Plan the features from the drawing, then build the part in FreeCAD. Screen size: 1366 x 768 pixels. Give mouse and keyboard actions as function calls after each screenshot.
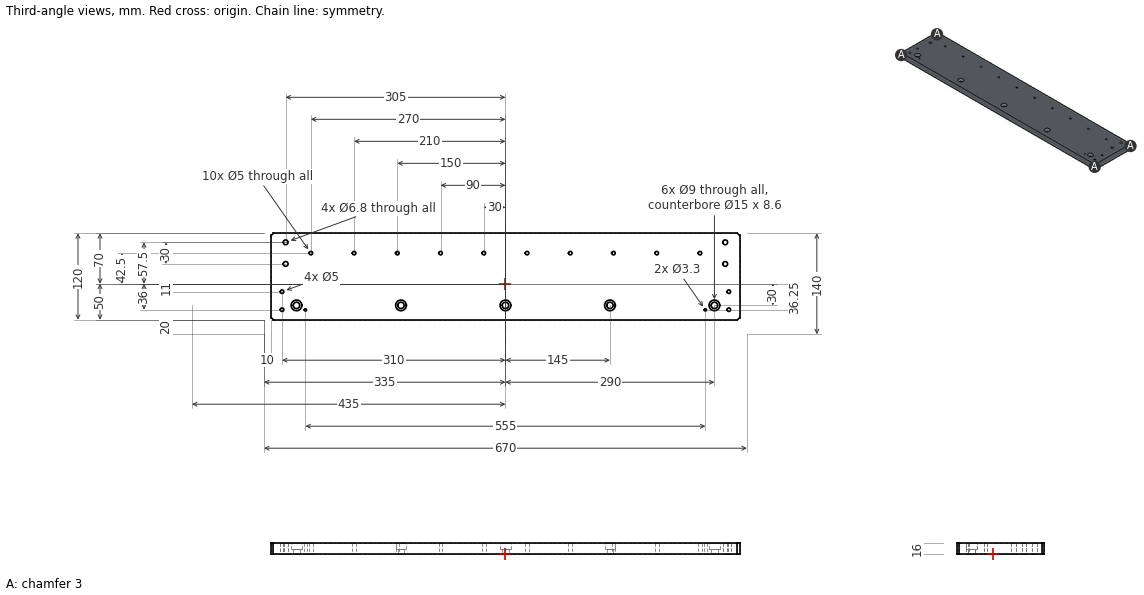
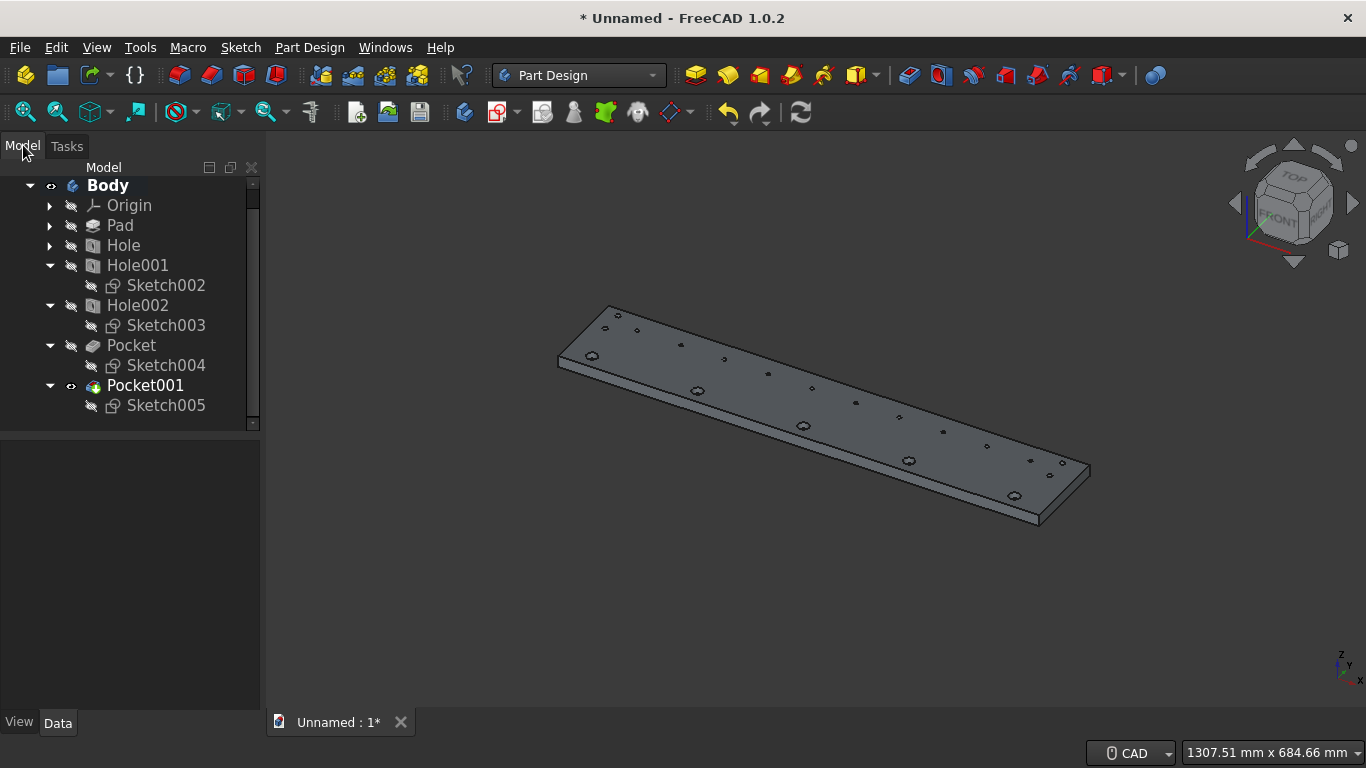
click(116, 386)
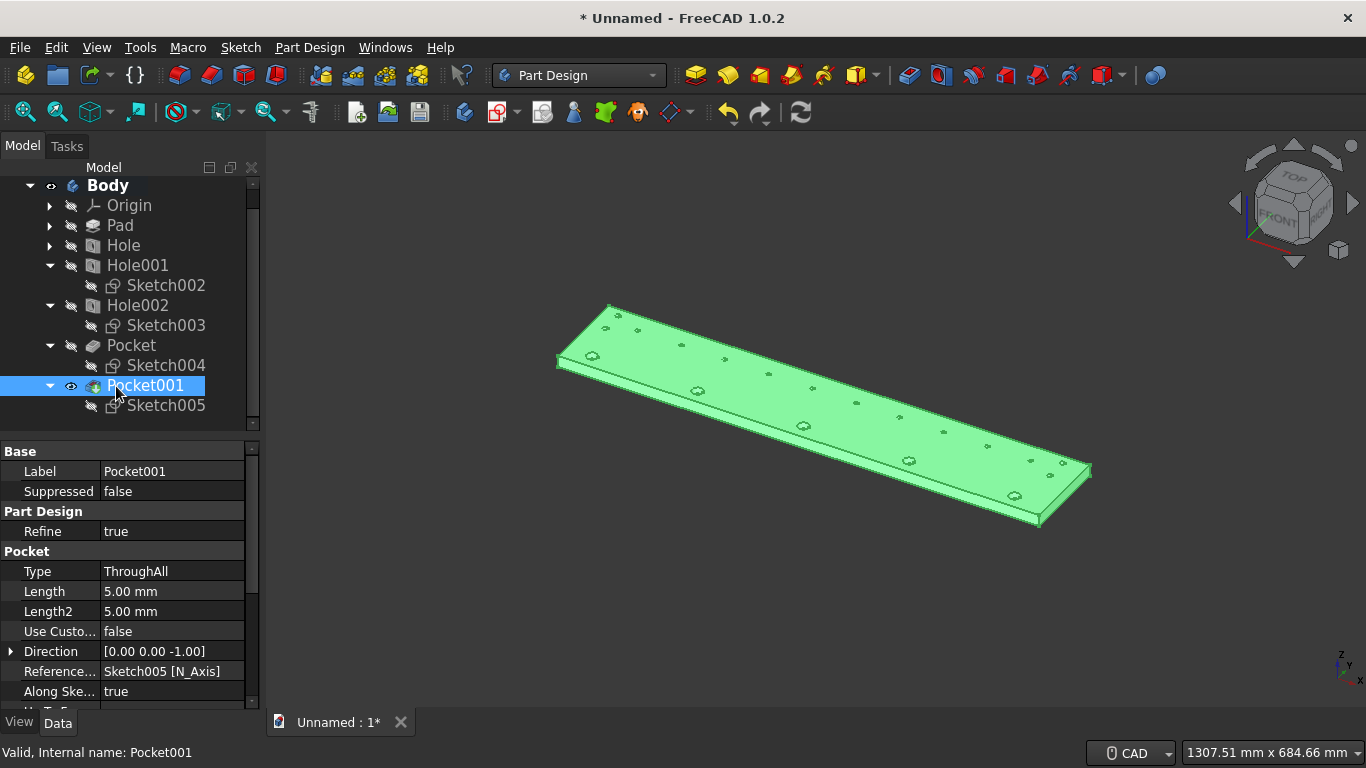
click(322, 76)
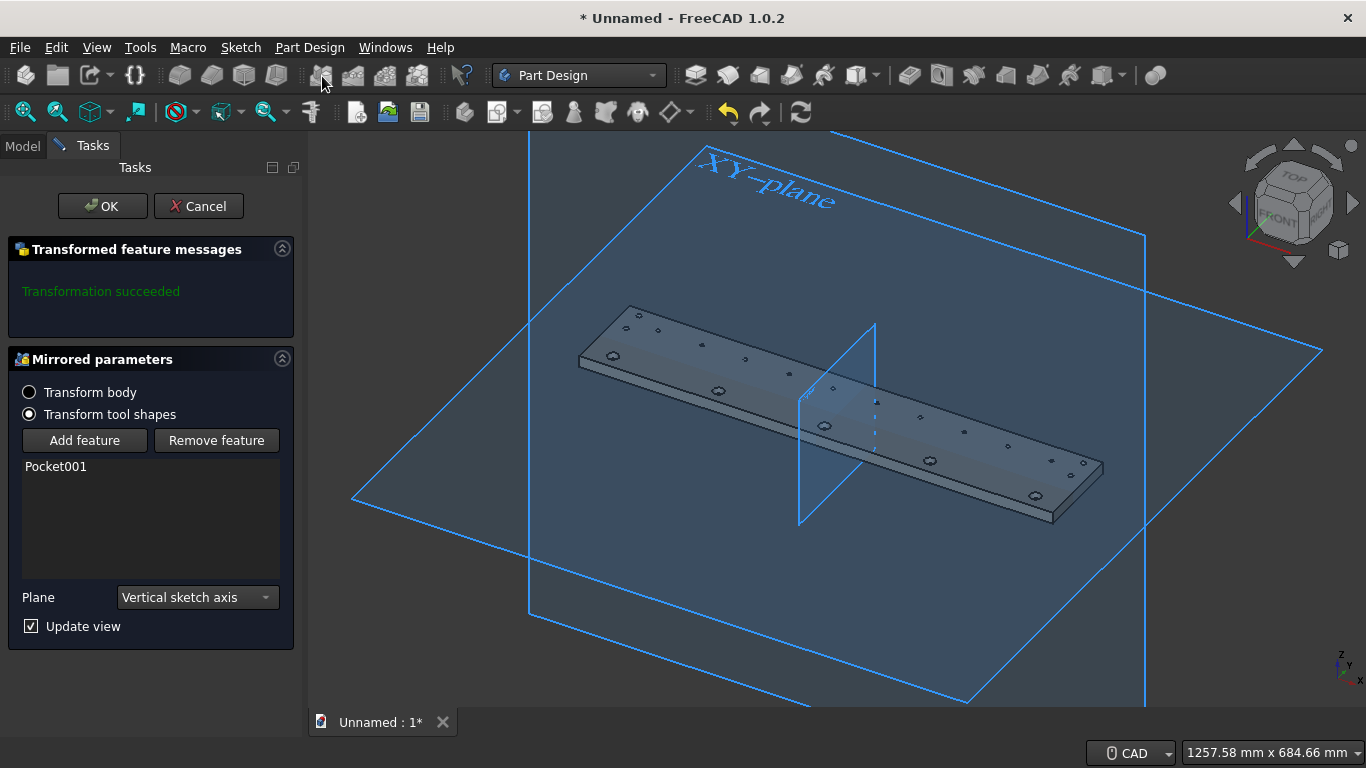
click(198, 598)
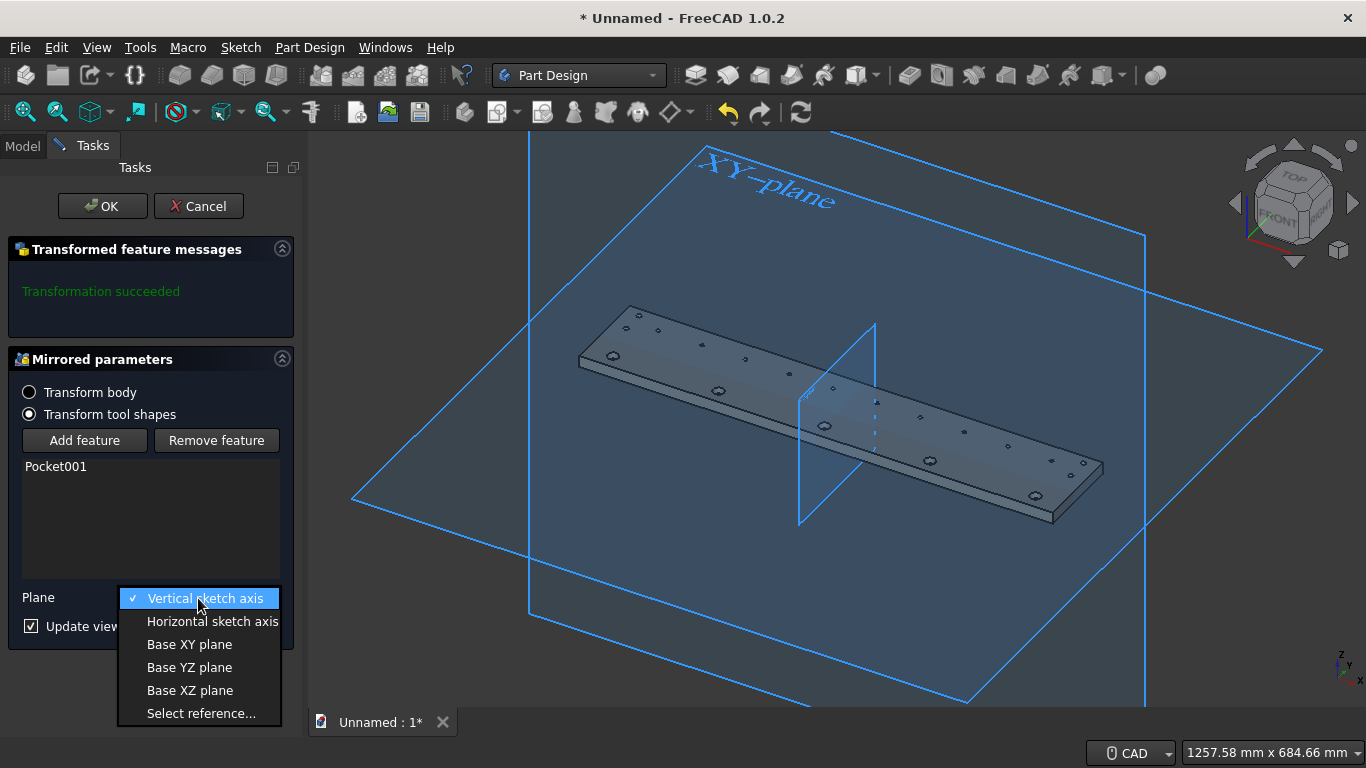
click(198, 668)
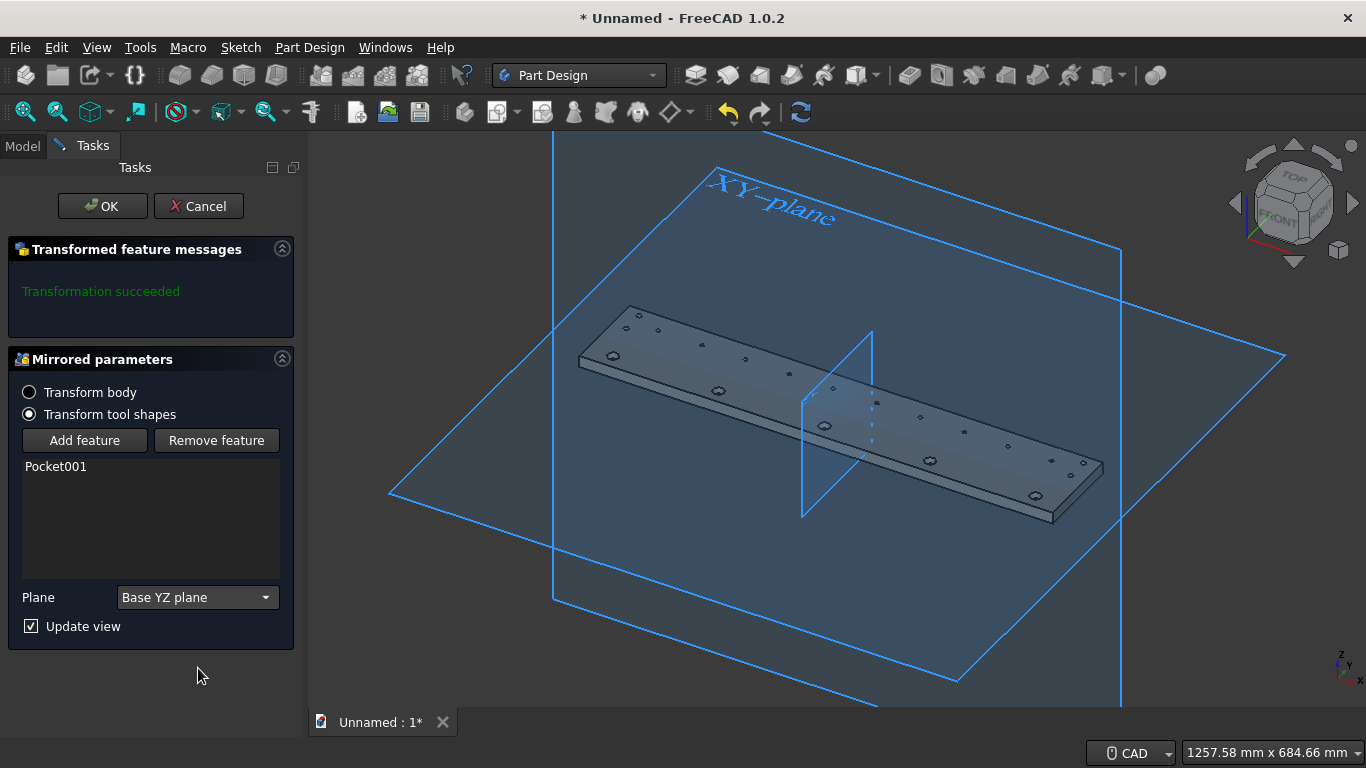
click(103, 206)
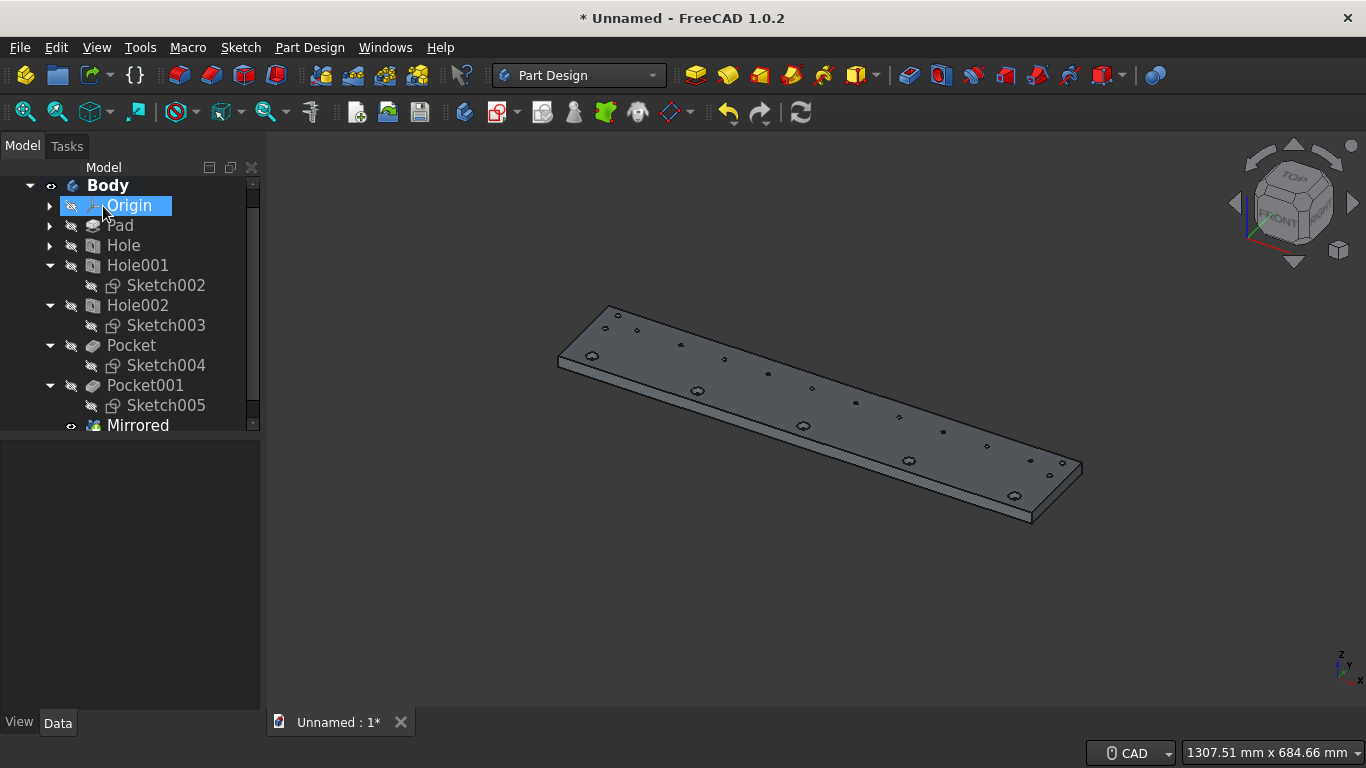
click(1032, 518)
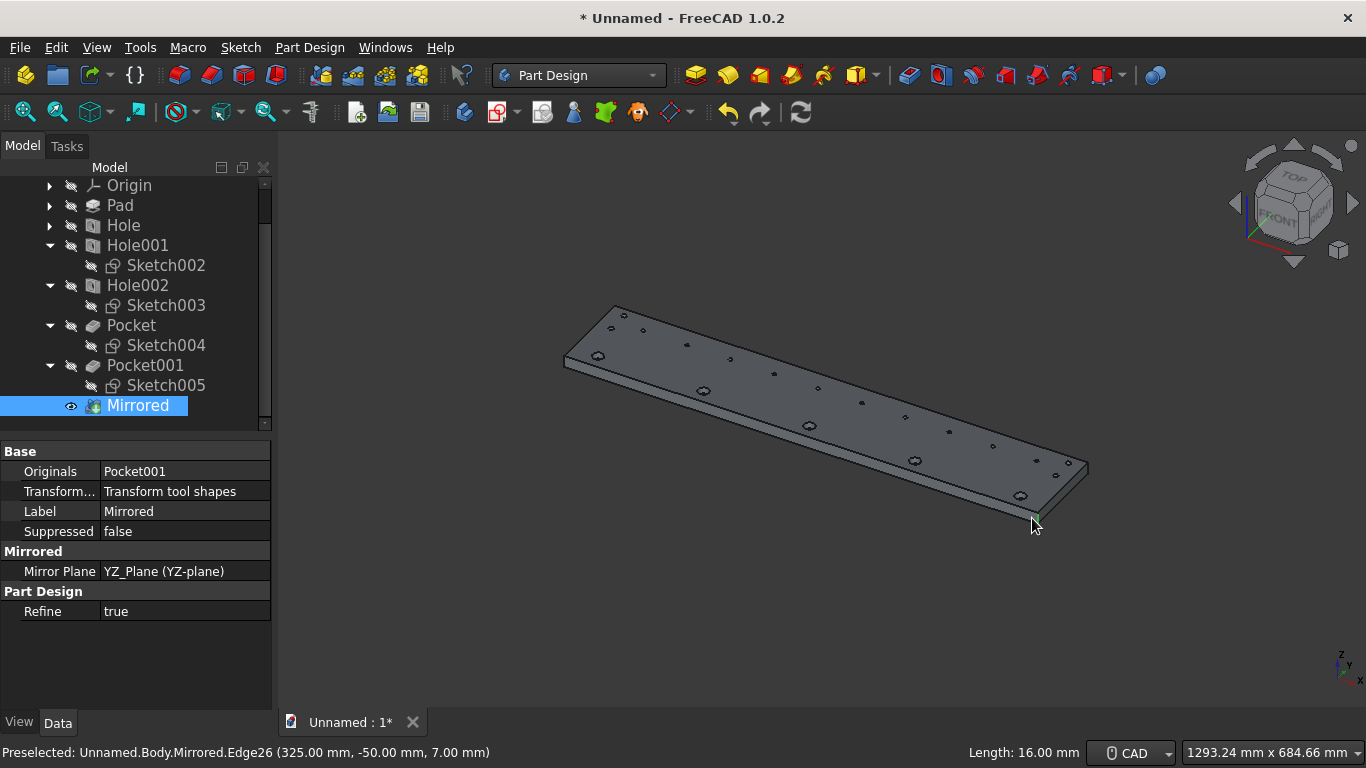
scroll(615, 310, up, 6)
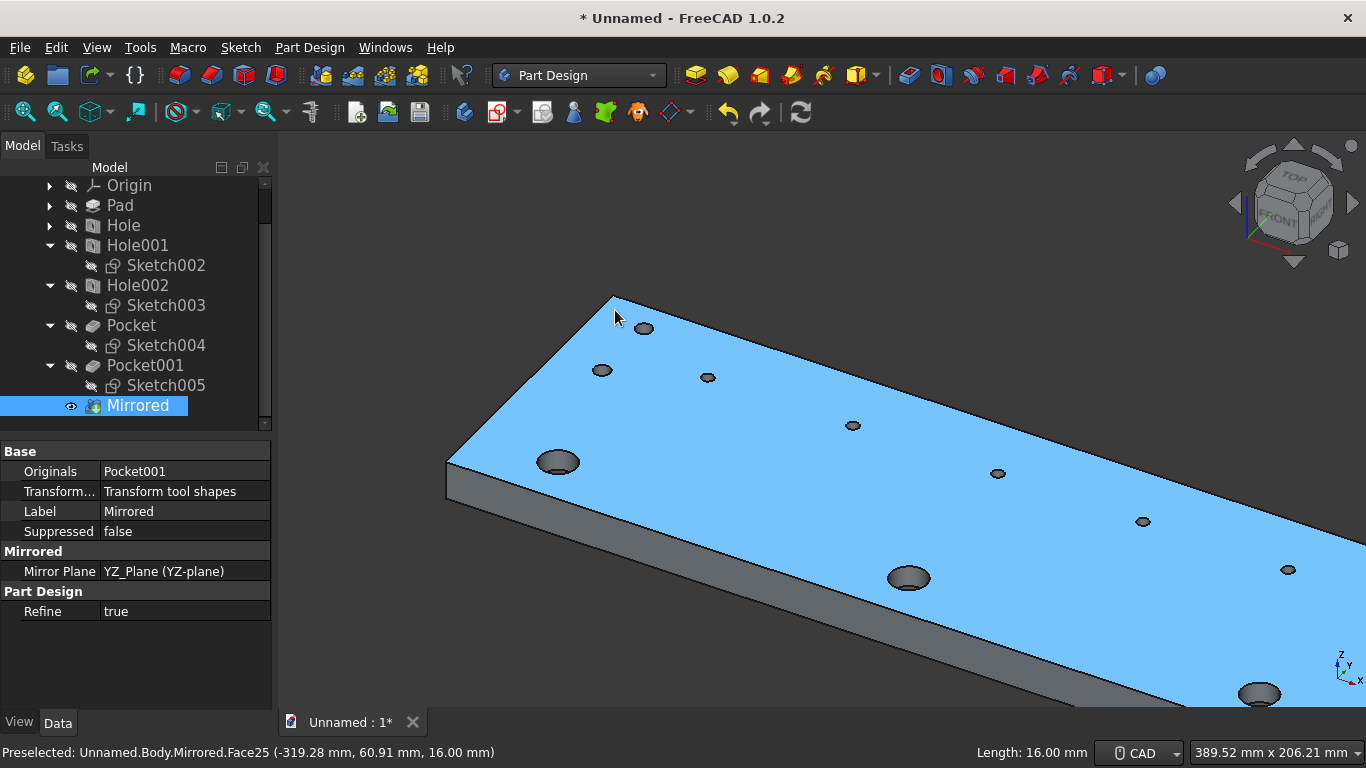
click(26, 112)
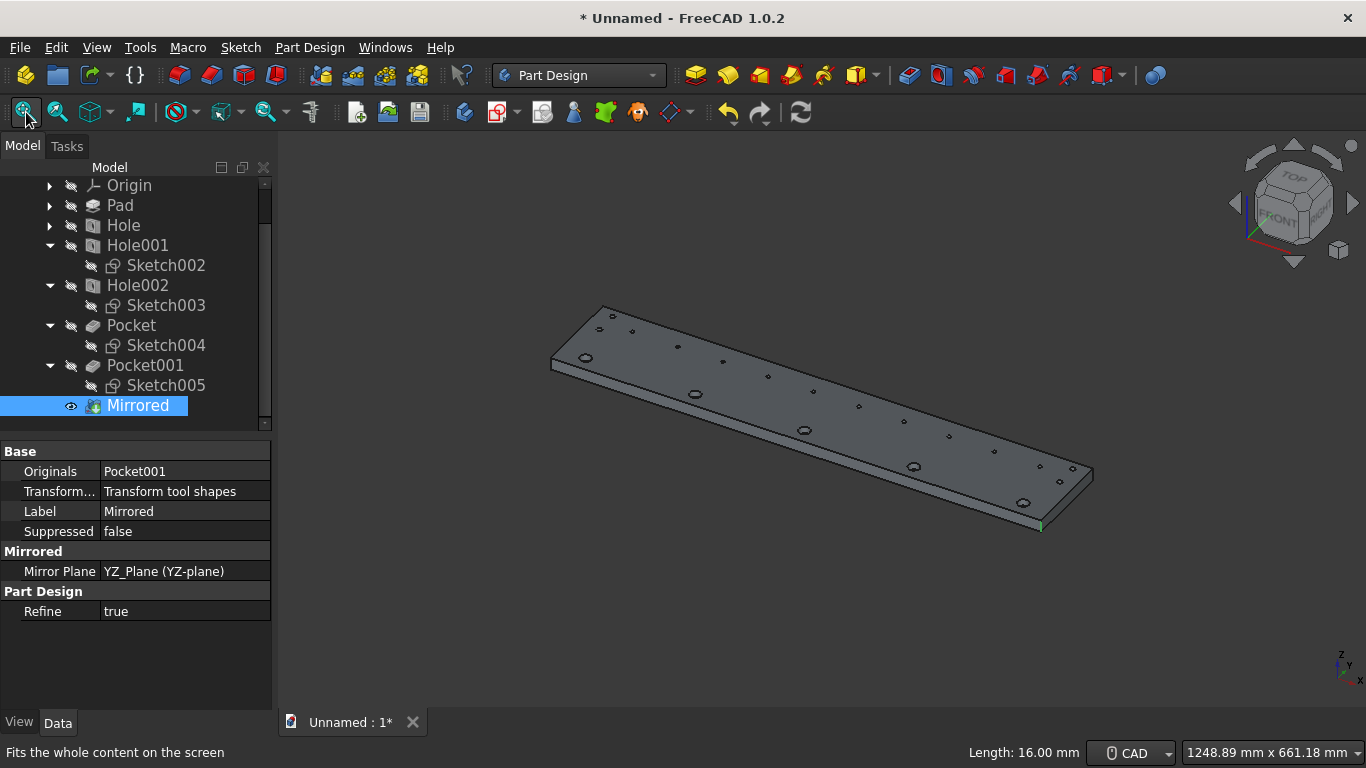
key(0)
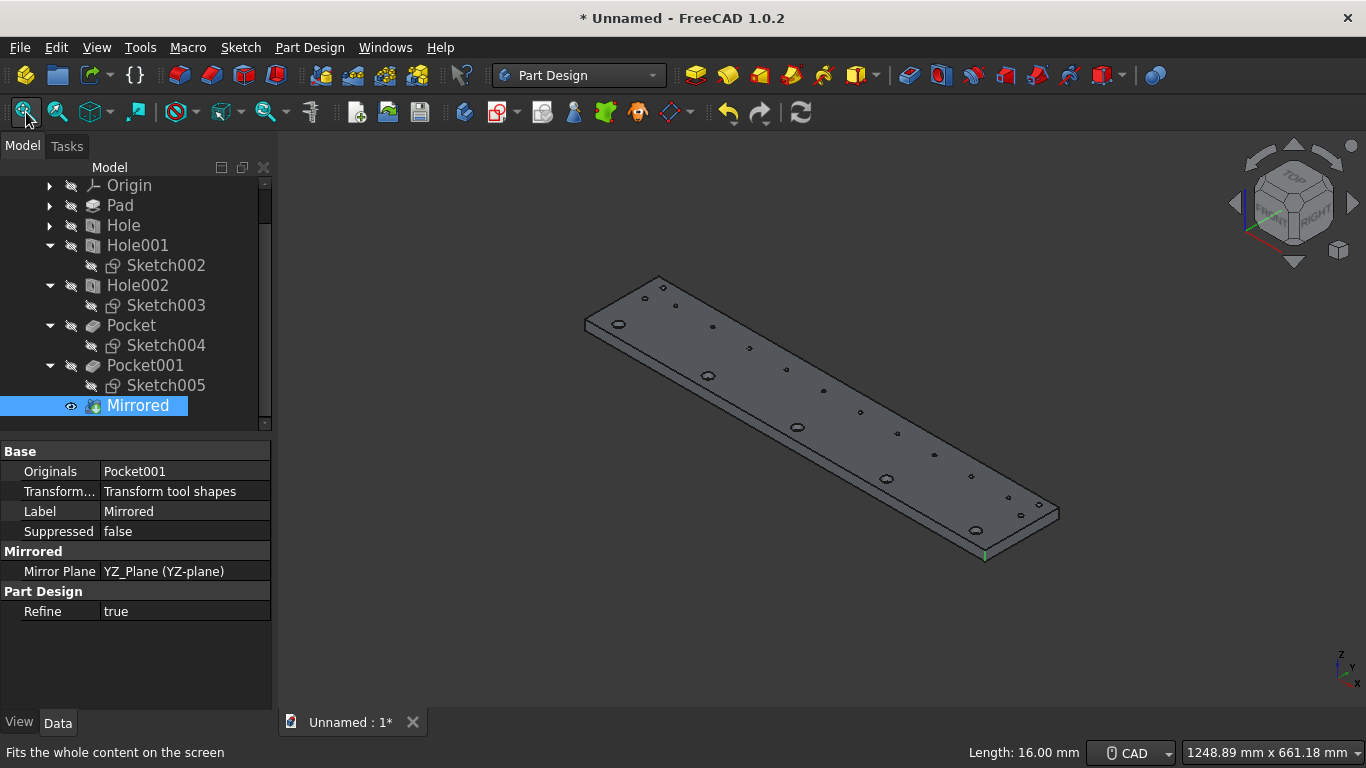
scroll(659, 281, up, 6)